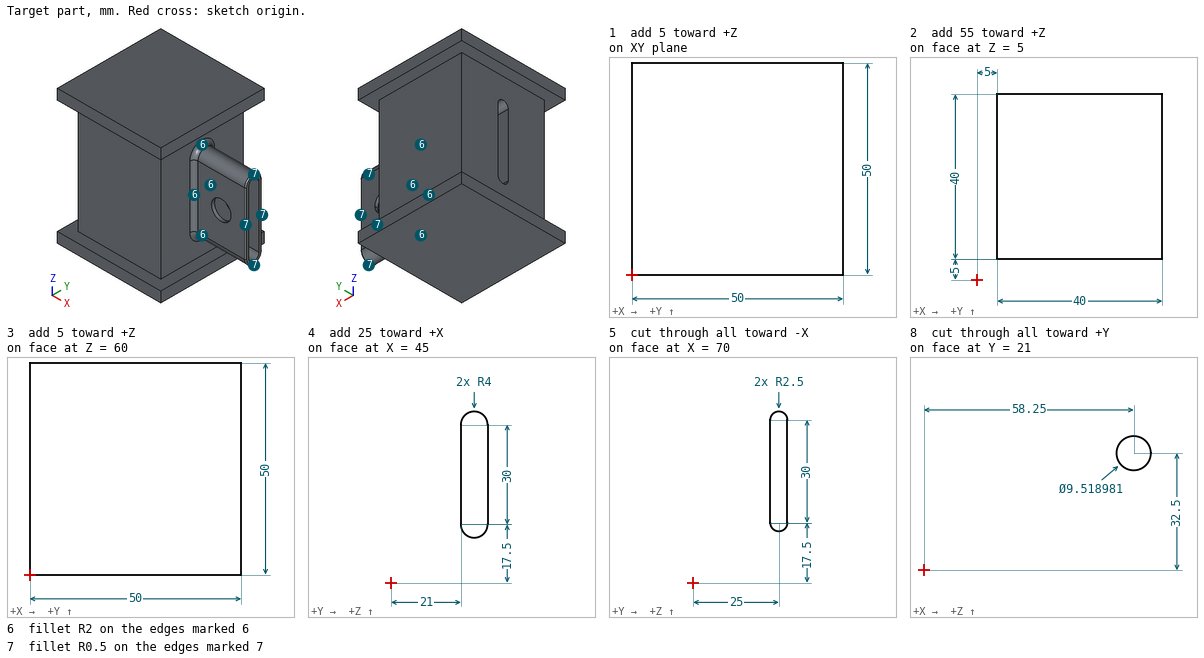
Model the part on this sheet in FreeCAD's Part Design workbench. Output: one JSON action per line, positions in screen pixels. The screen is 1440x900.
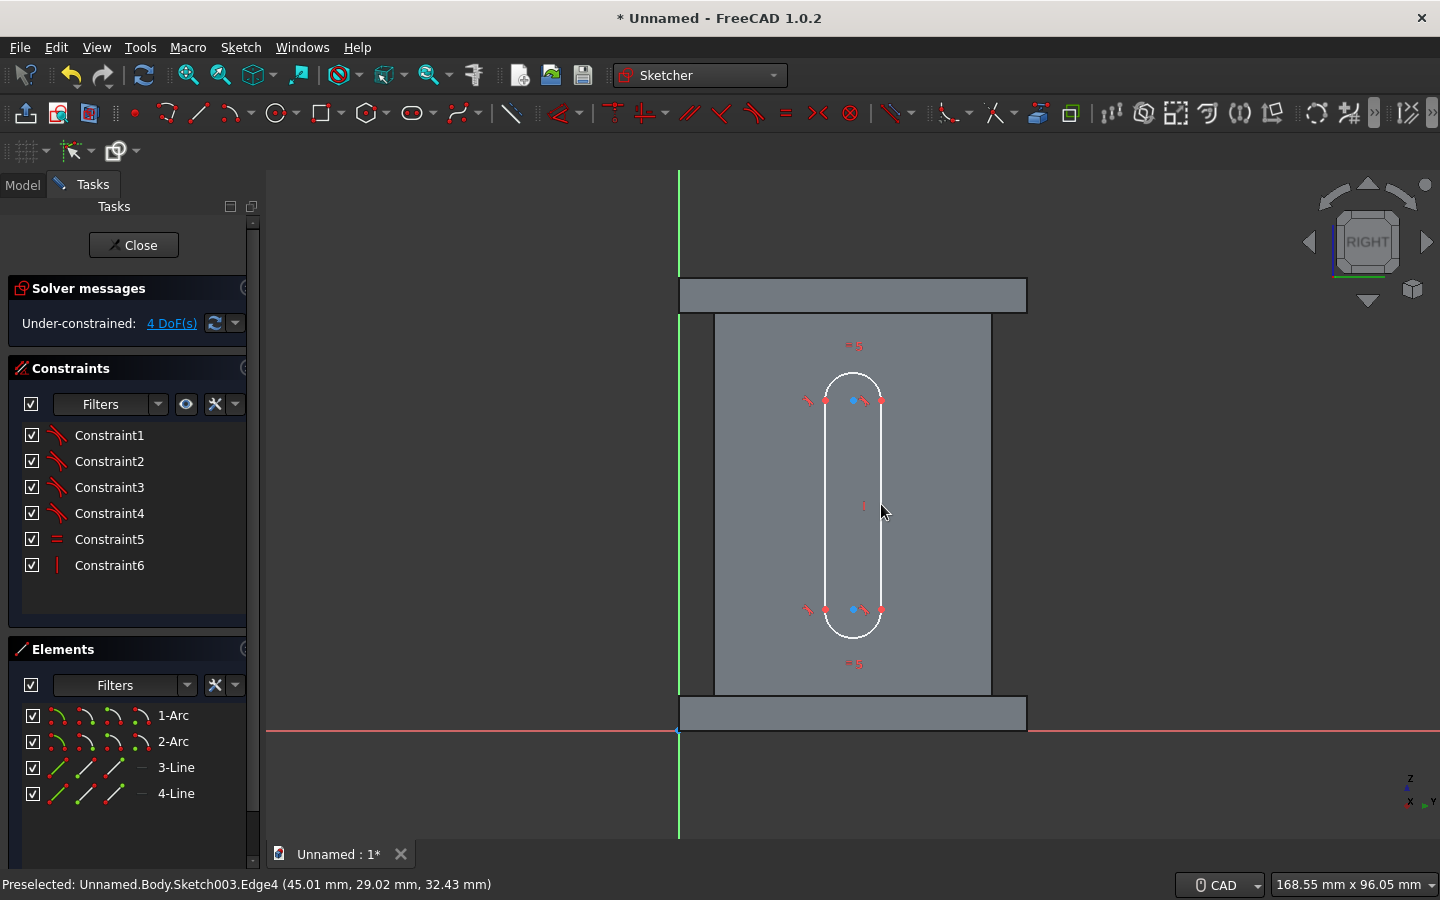
{"action": "left_click", "coordinate": [558, 114]}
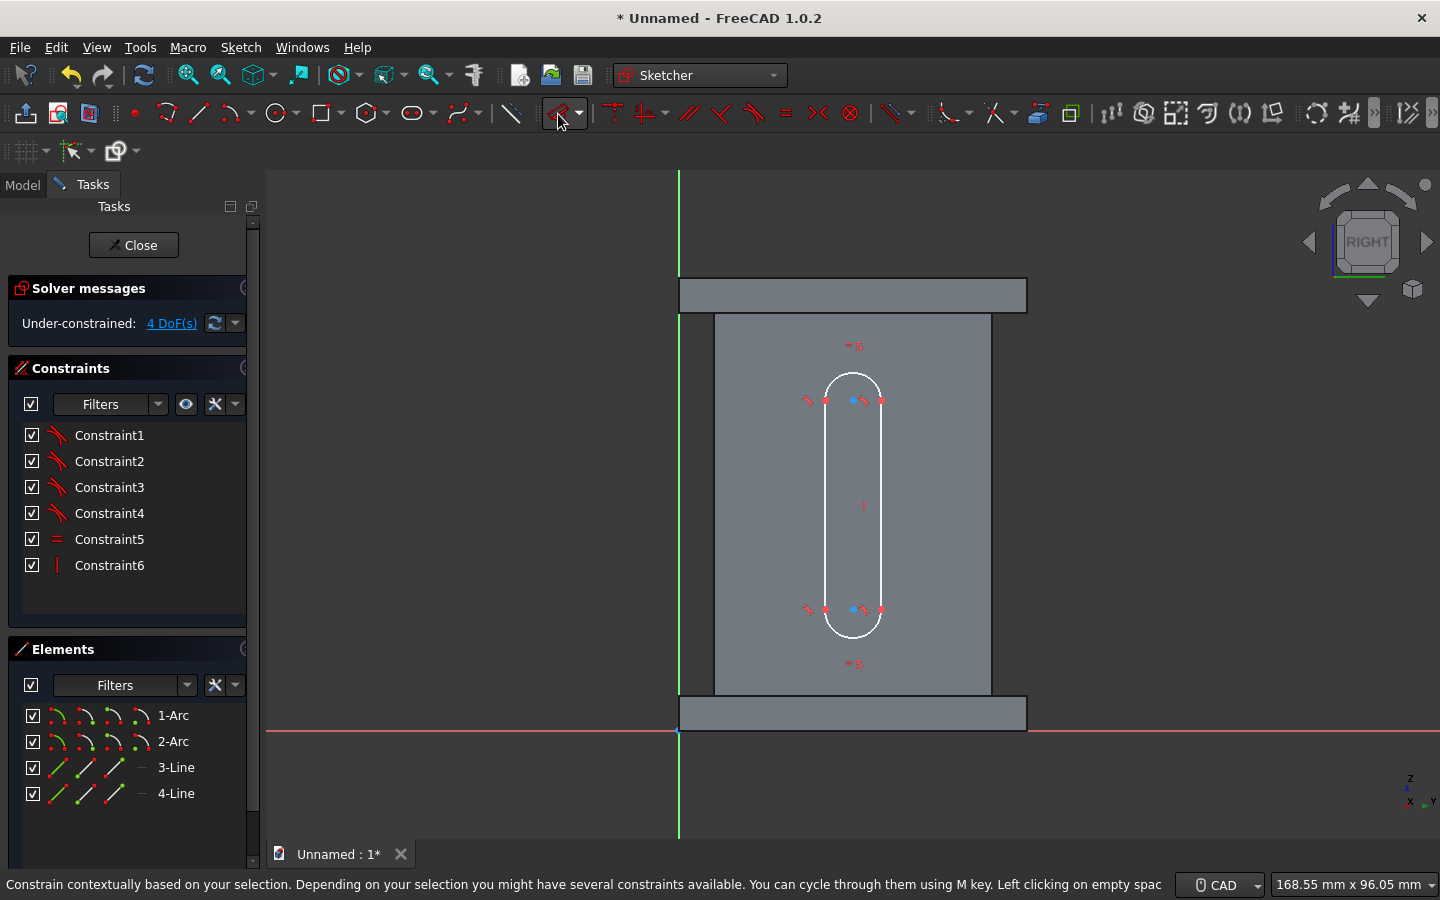
{"action": "scroll", "coordinate": [837, 633], "scroll_direction": "up", "scroll_amount": 2}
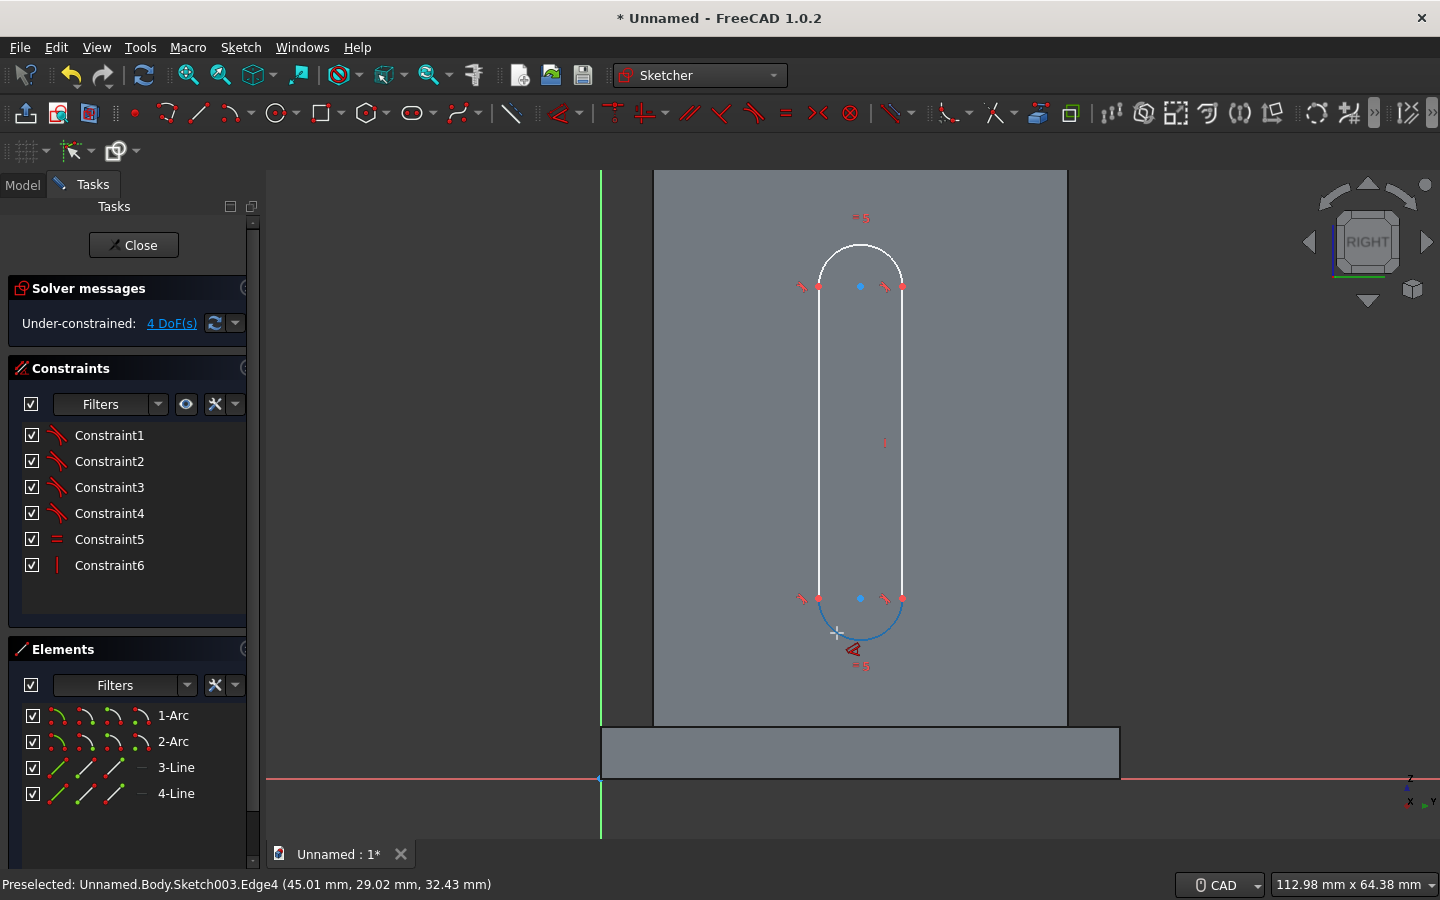
{"action": "left_click", "coordinate": [836, 632]}
{"action": "left_click", "coordinate": [817, 658]}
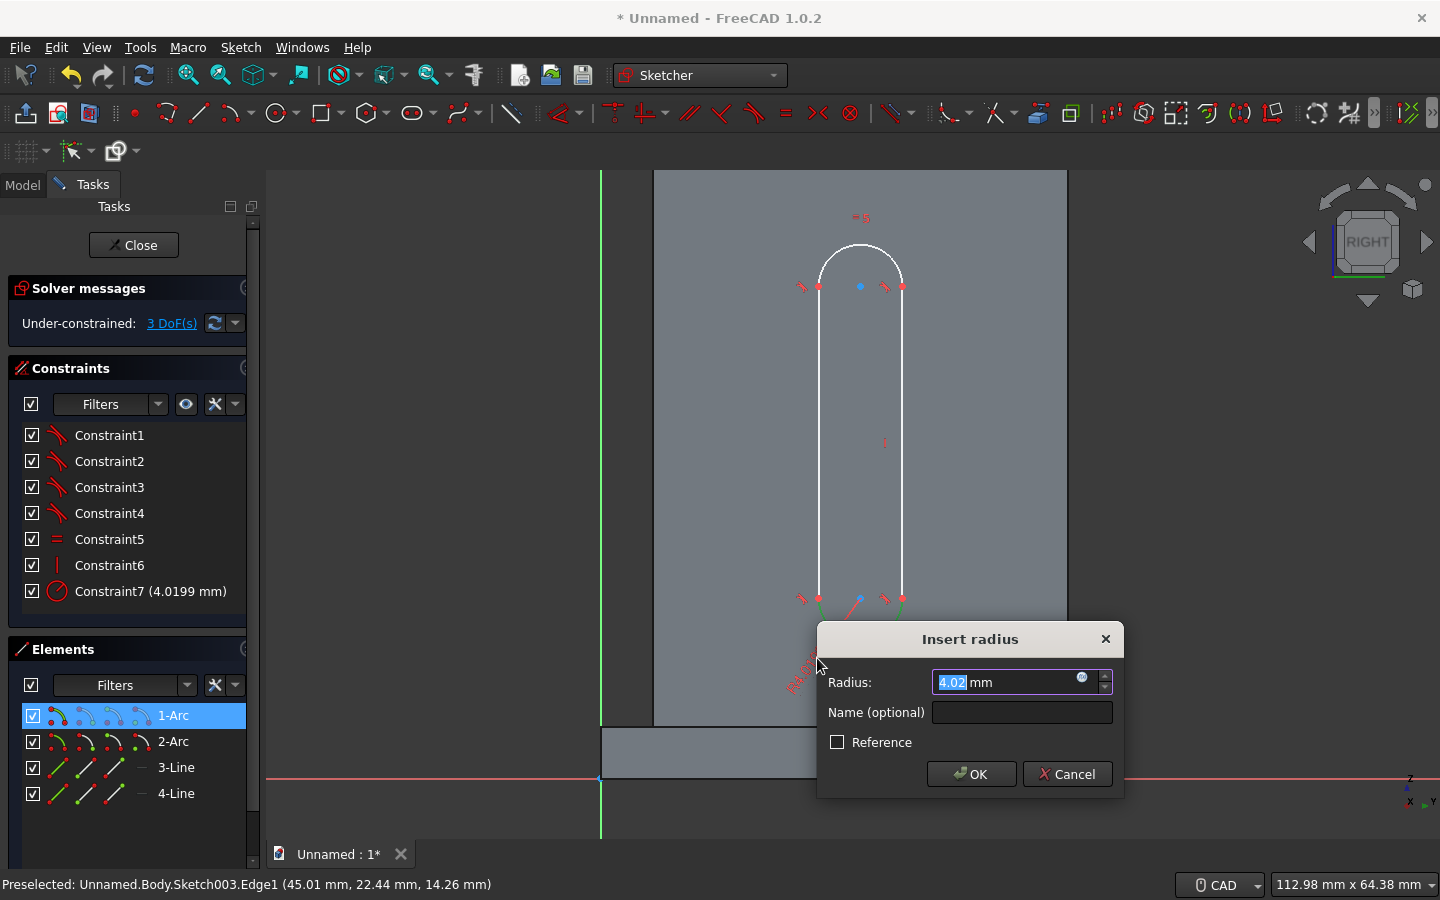
{"action": "type", "text": "4"}
{"action": "key", "text": "Return"}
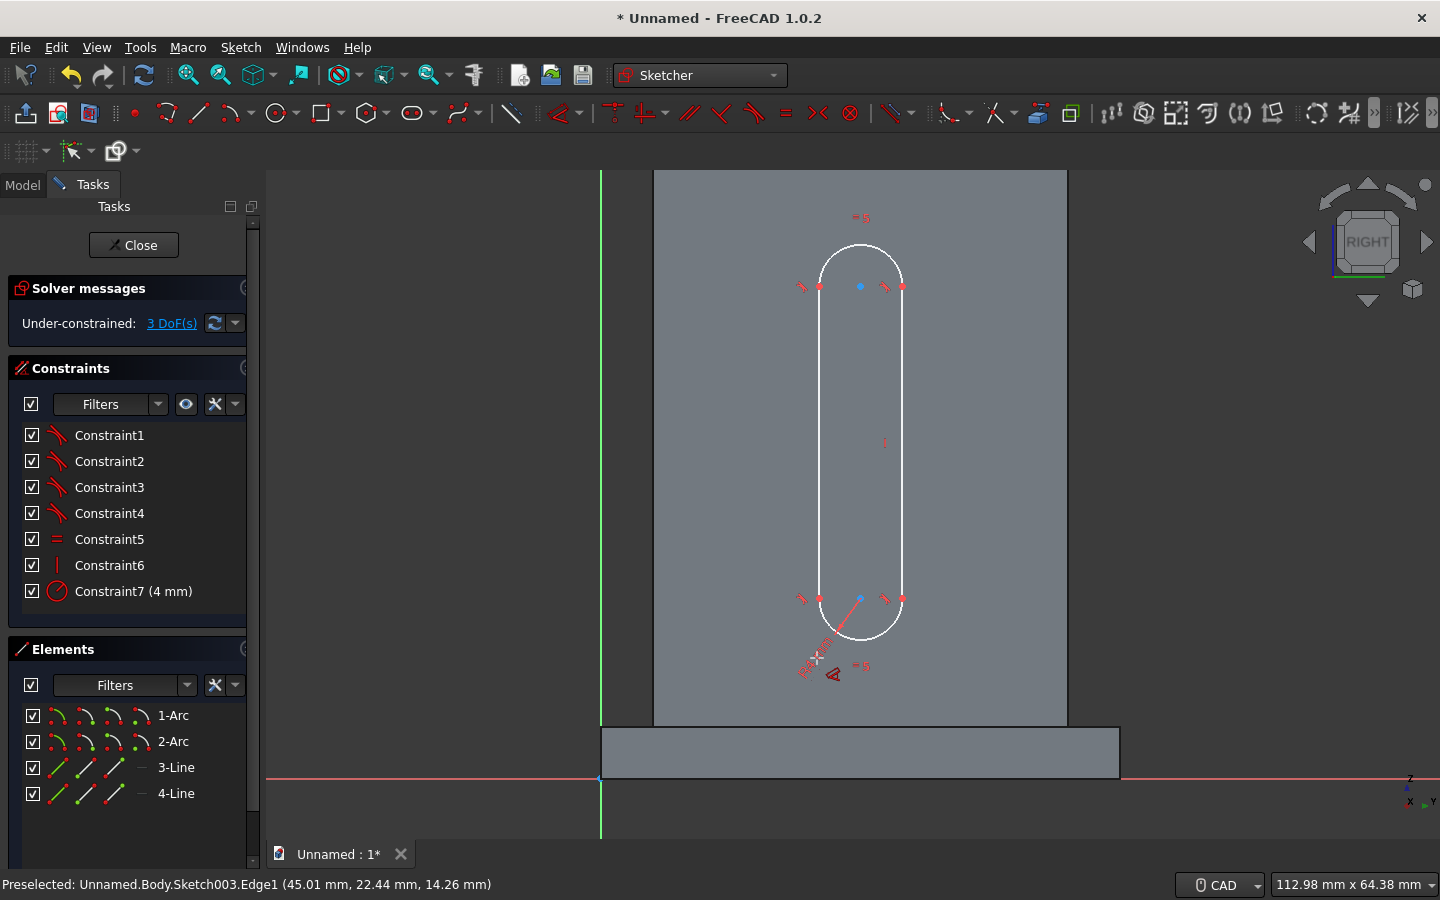
{"action": "left_click", "coordinate": [819, 505]}
{"action": "left_click", "coordinate": [853, 442]}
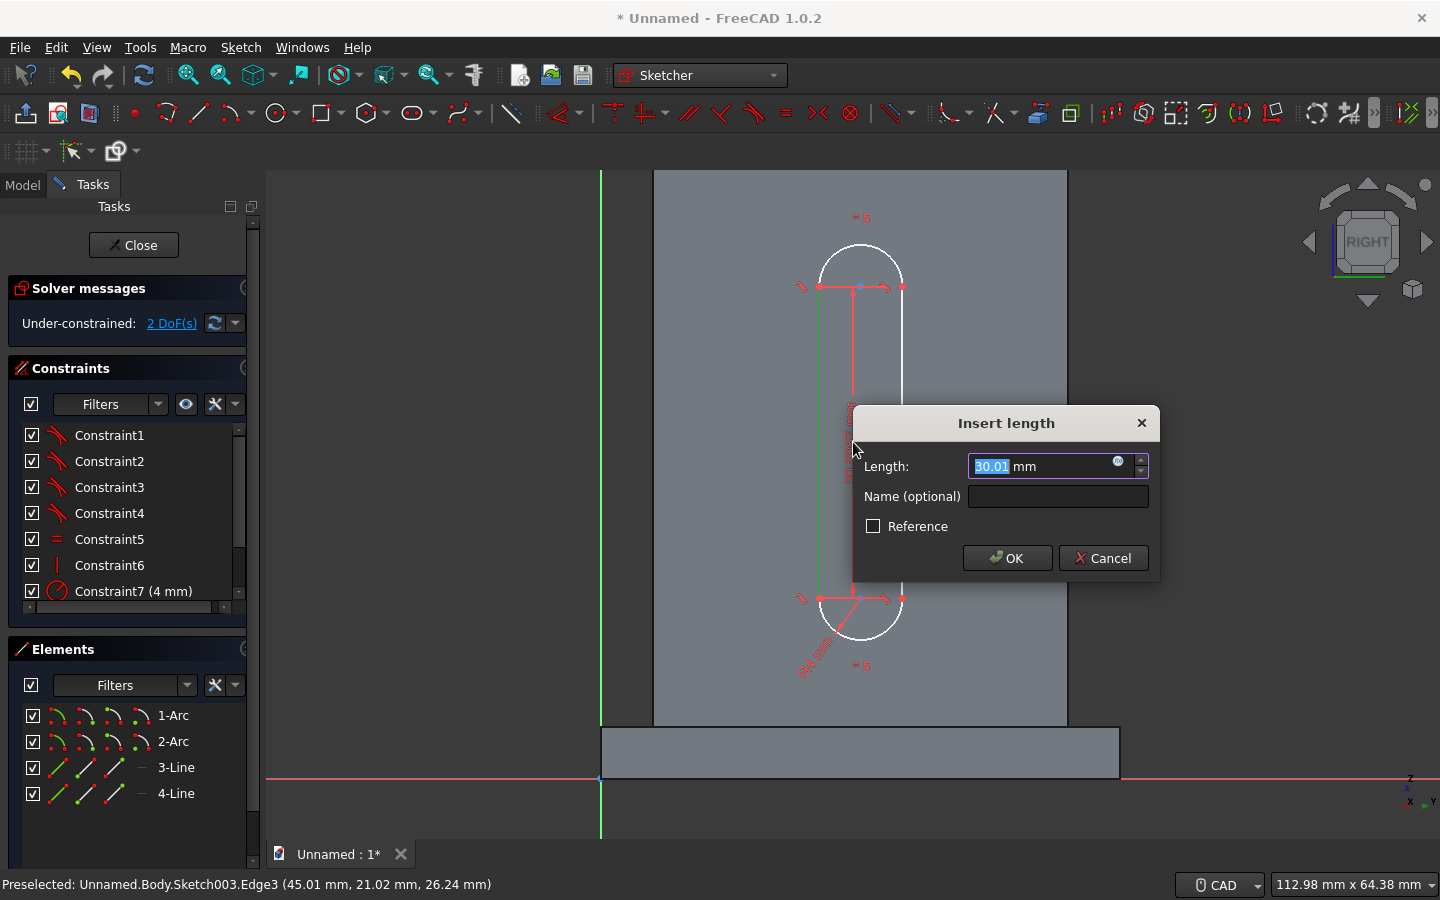
{"action": "type", "text": "30"}
{"action": "key", "text": "Return"}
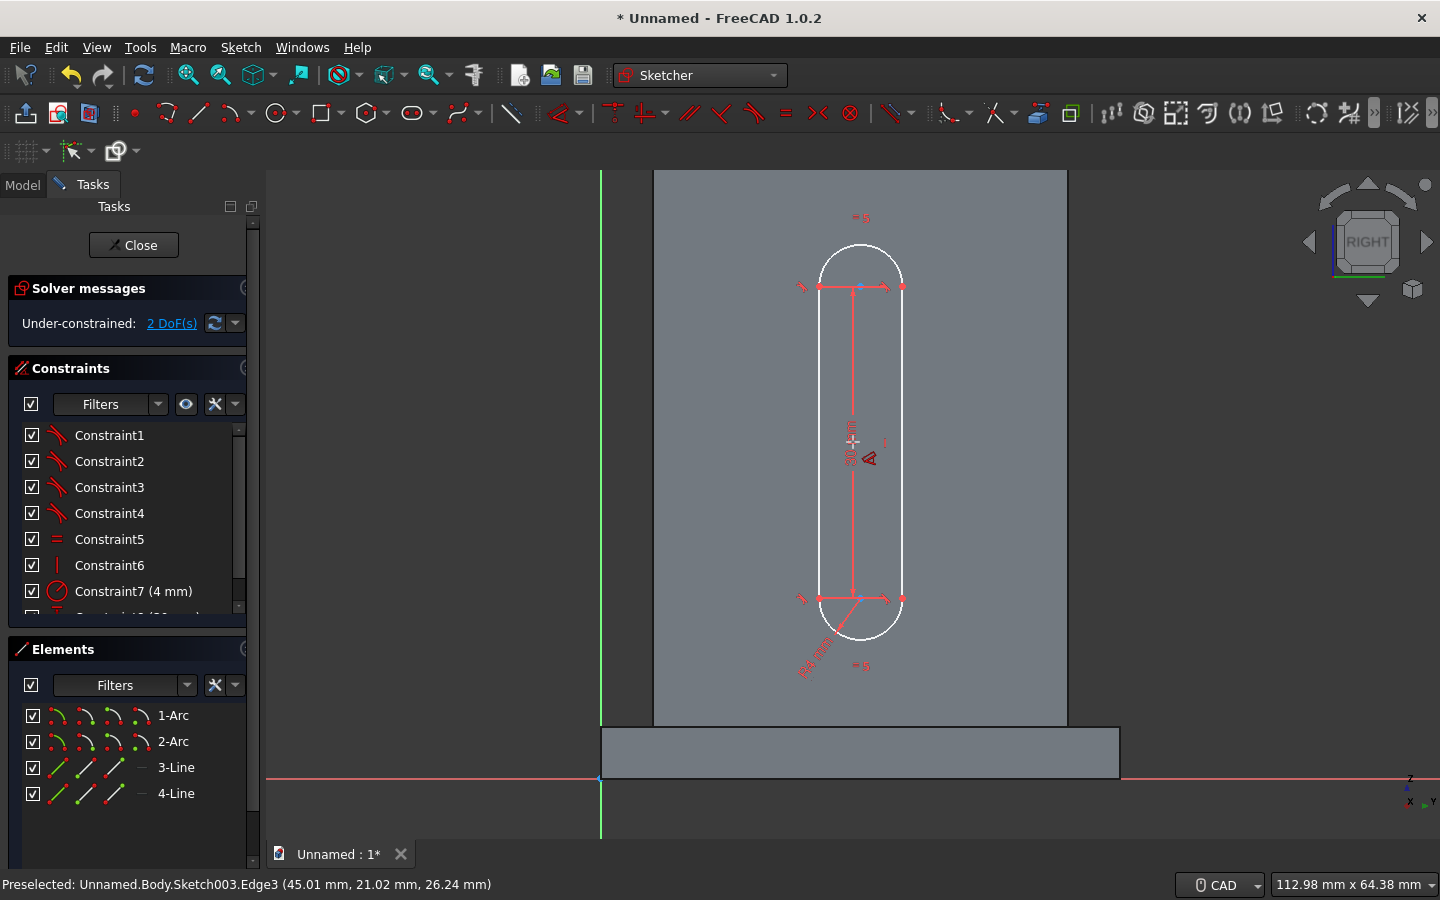
{"action": "left_click", "coordinate": [819, 598]}
{"action": "left_click", "coordinate": [710, 564]}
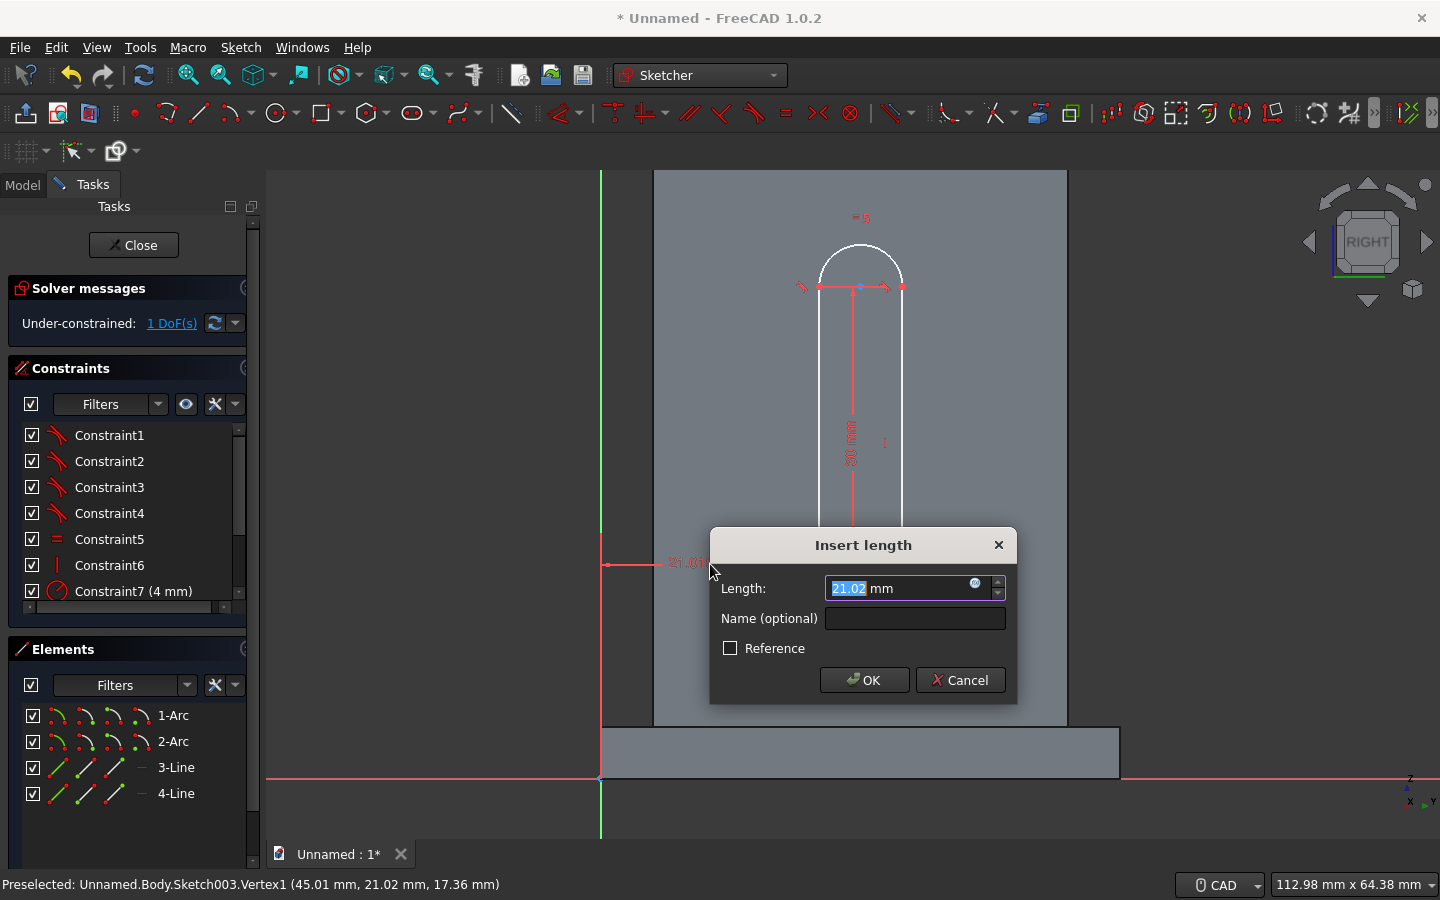
{"action": "type", "text": "21"}
{"action": "key", "text": "Return"}